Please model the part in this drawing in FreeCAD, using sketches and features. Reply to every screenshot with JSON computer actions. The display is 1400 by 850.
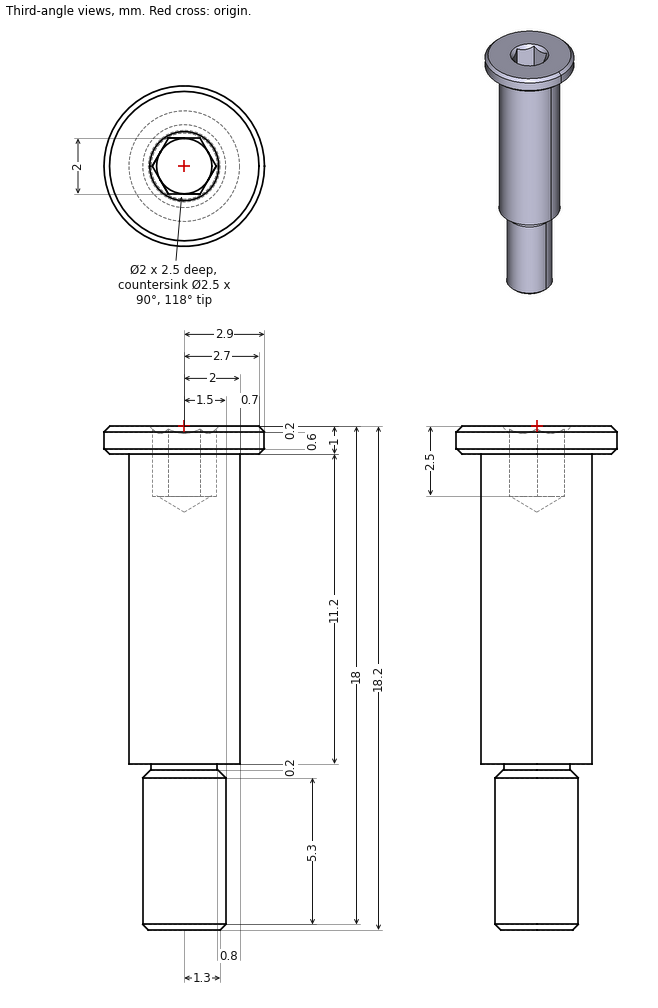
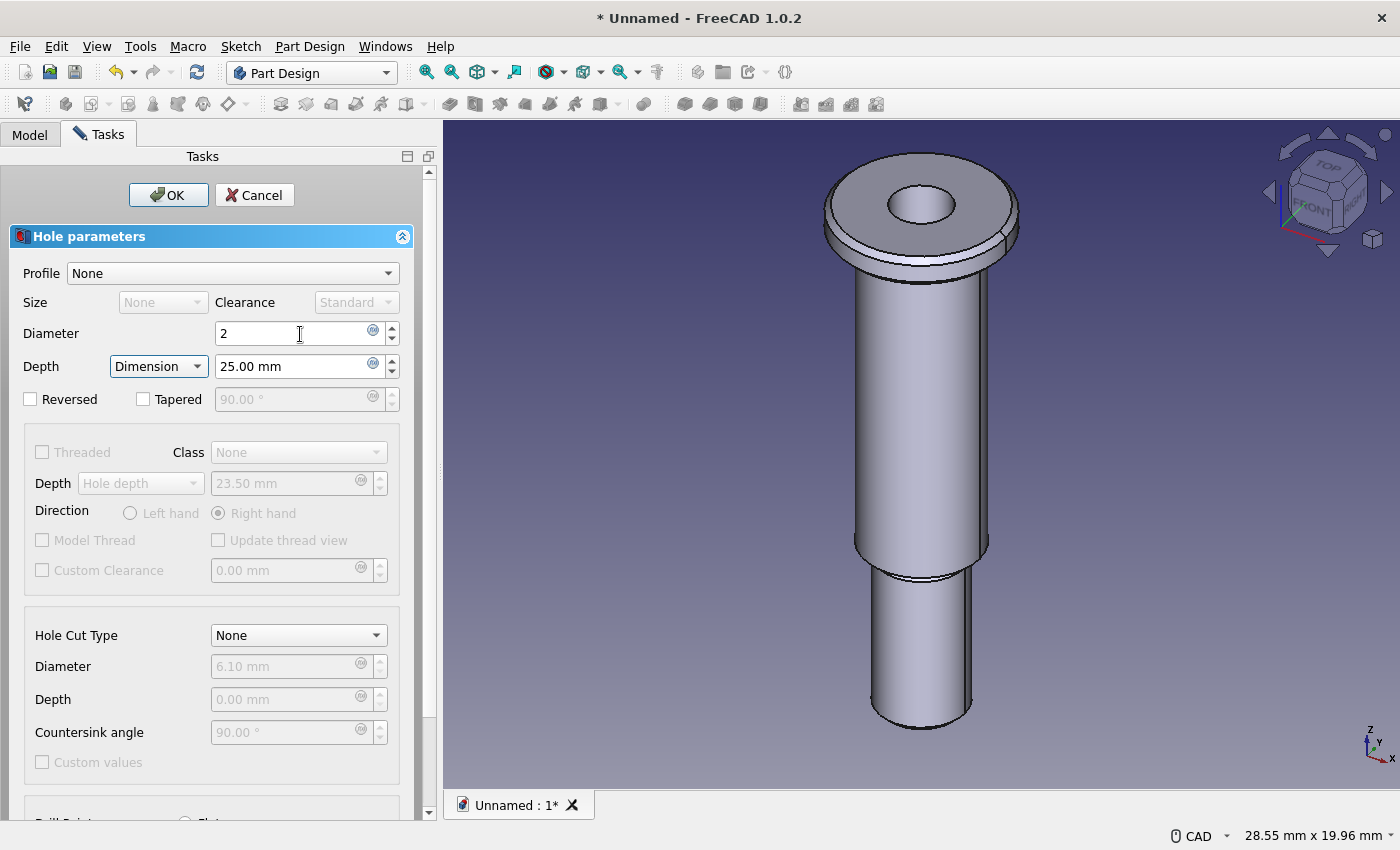
{"action": "triple_click", "coordinate": [300, 366]}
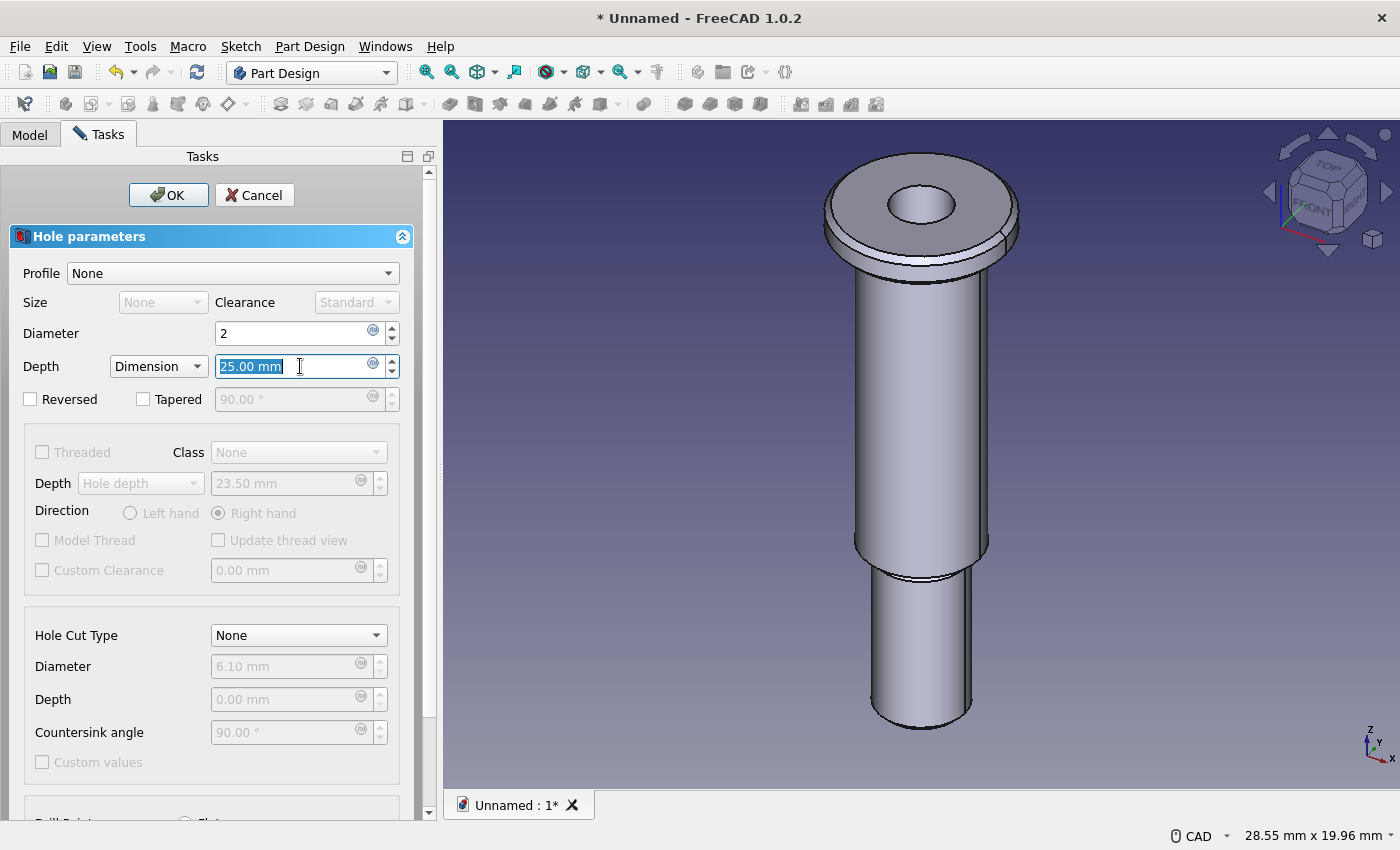
{"action": "type", "text": "2.5"}
{"action": "key", "text": "Tab"}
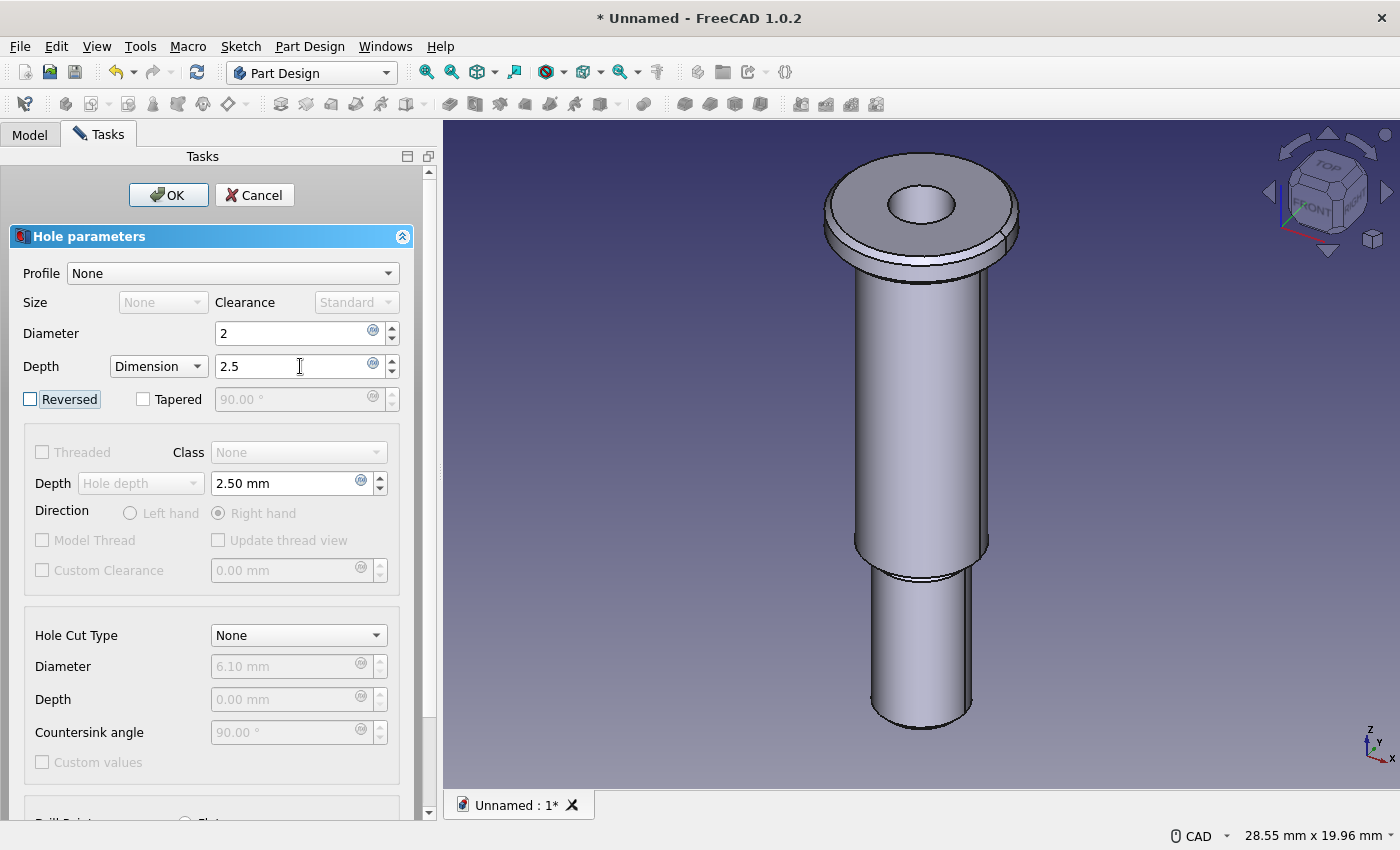
{"action": "left_click", "coordinate": [300, 636]}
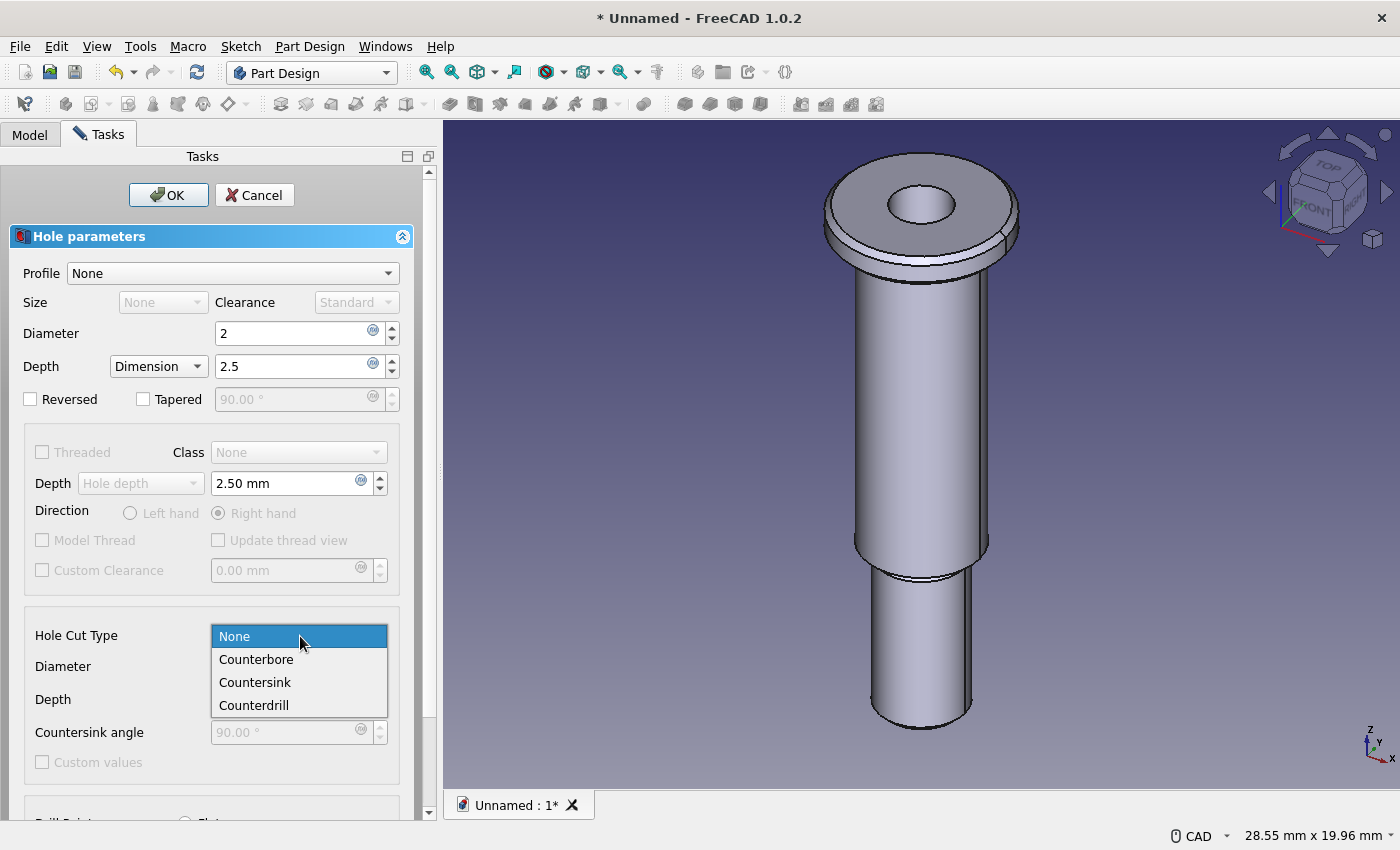
{"action": "left_click", "coordinate": [298, 682]}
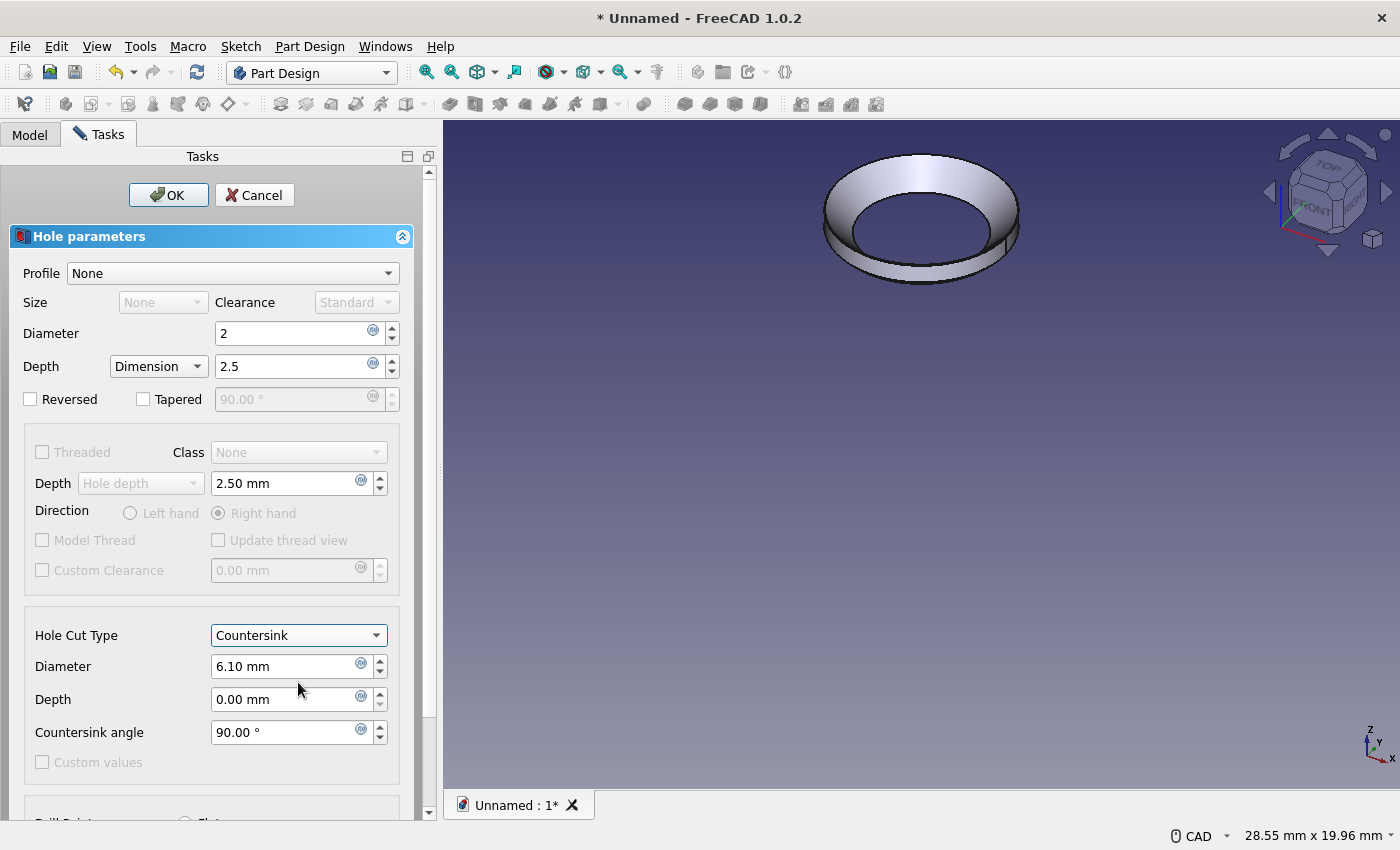
{"action": "triple_click", "coordinate": [292, 666]}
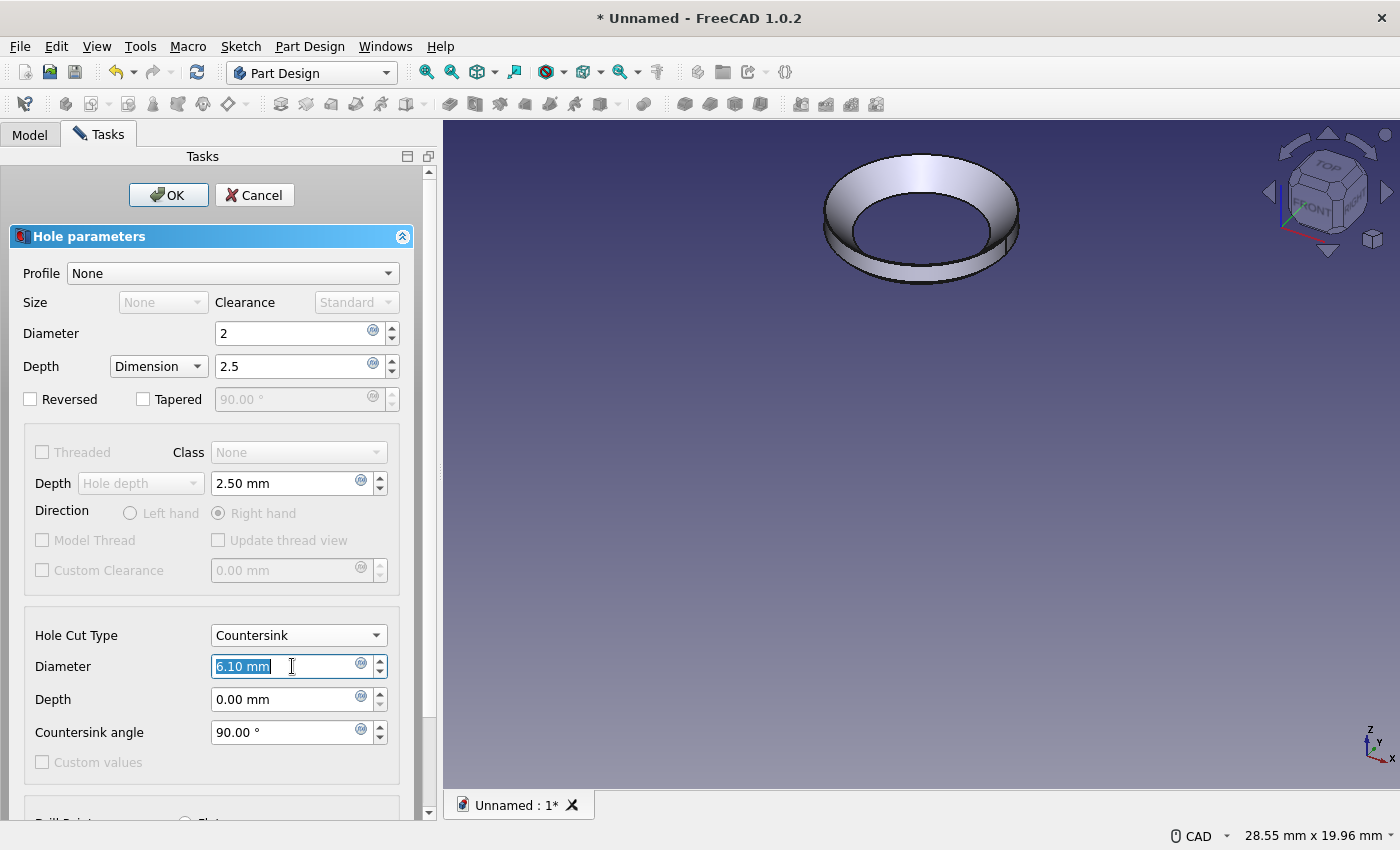
{"action": "type", "text": "2.5"}
{"action": "key", "text": "Tab"}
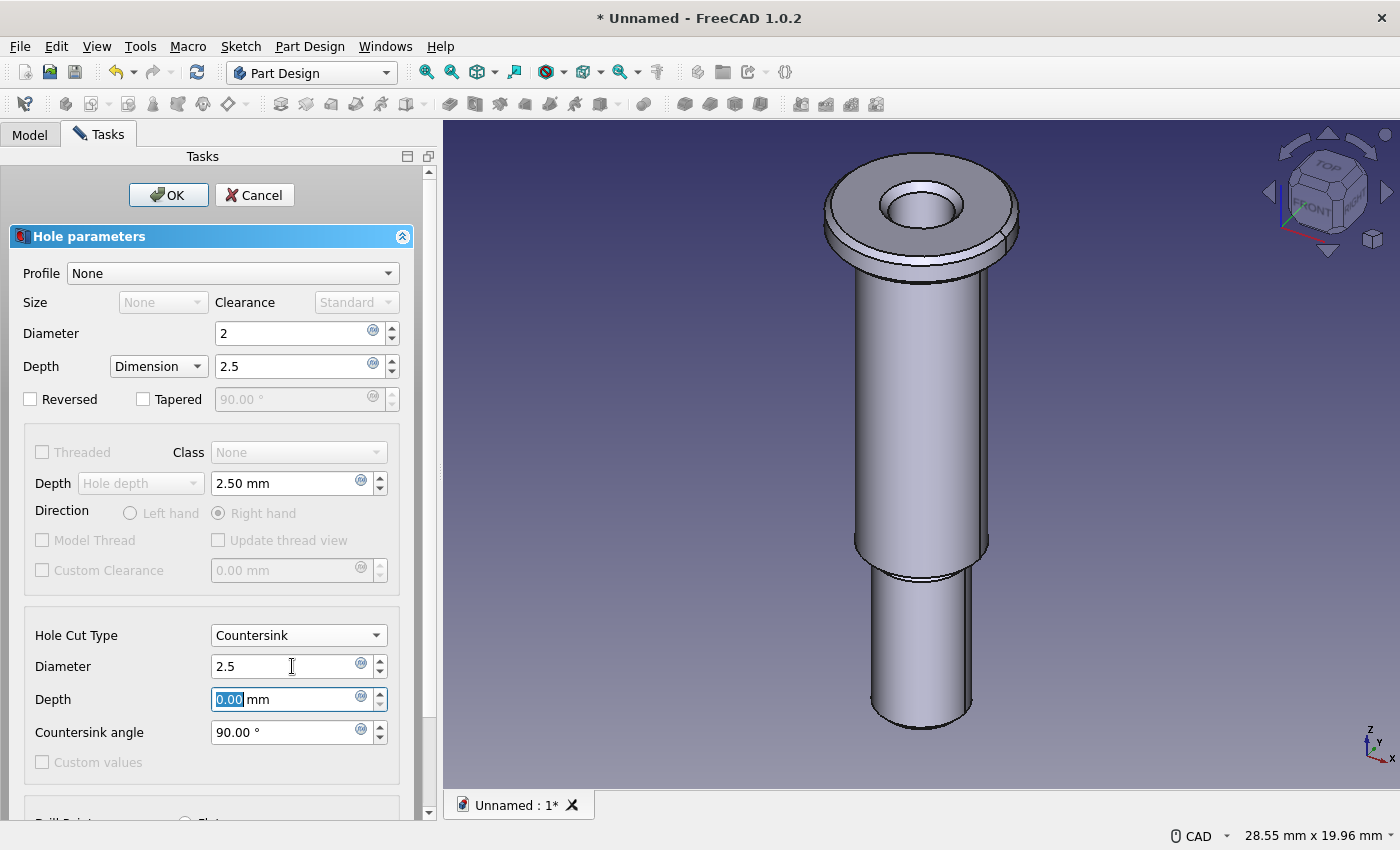
{"action": "left_click", "coordinate": [169, 195]}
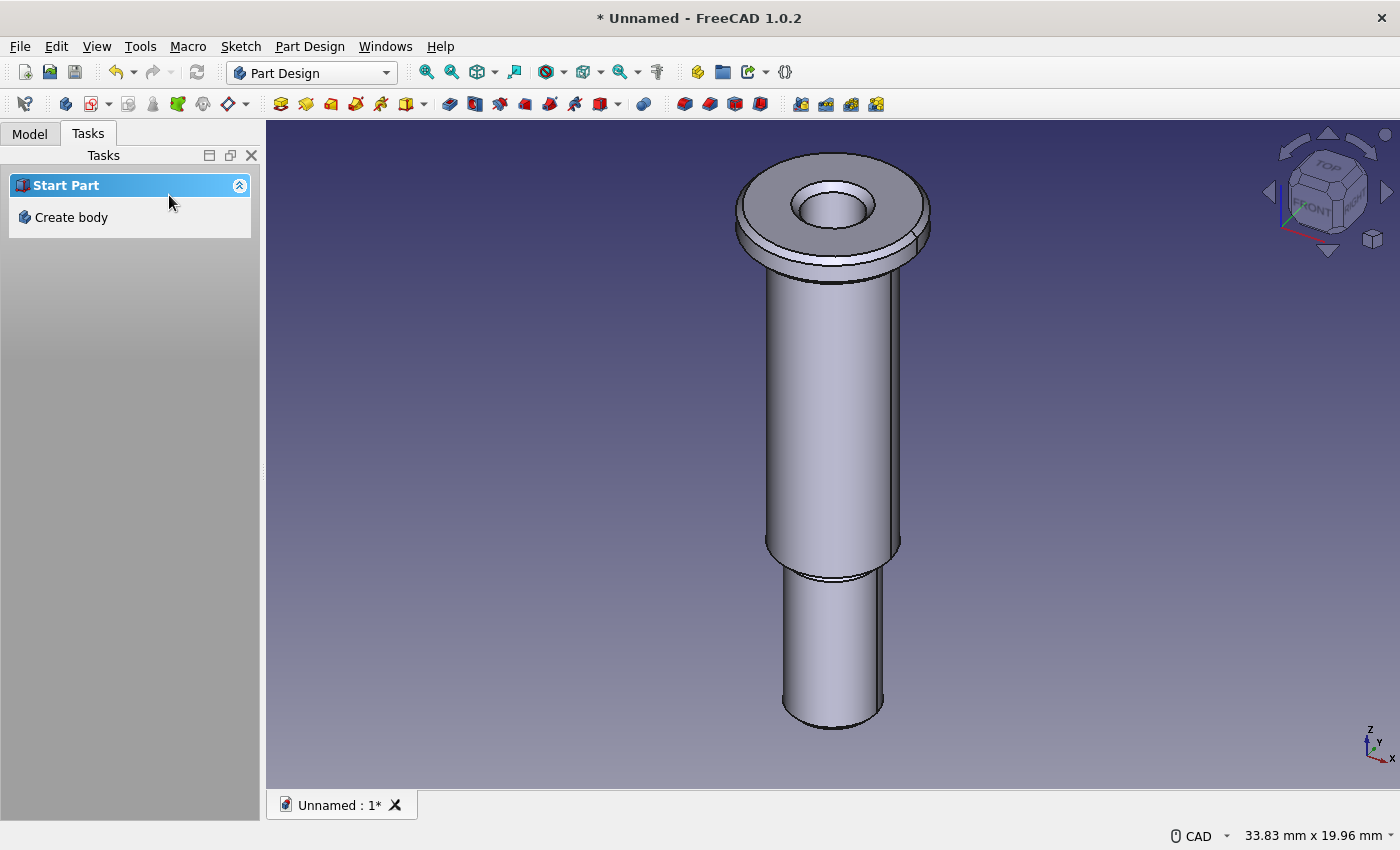
{"action": "left_click", "coordinate": [90, 104]}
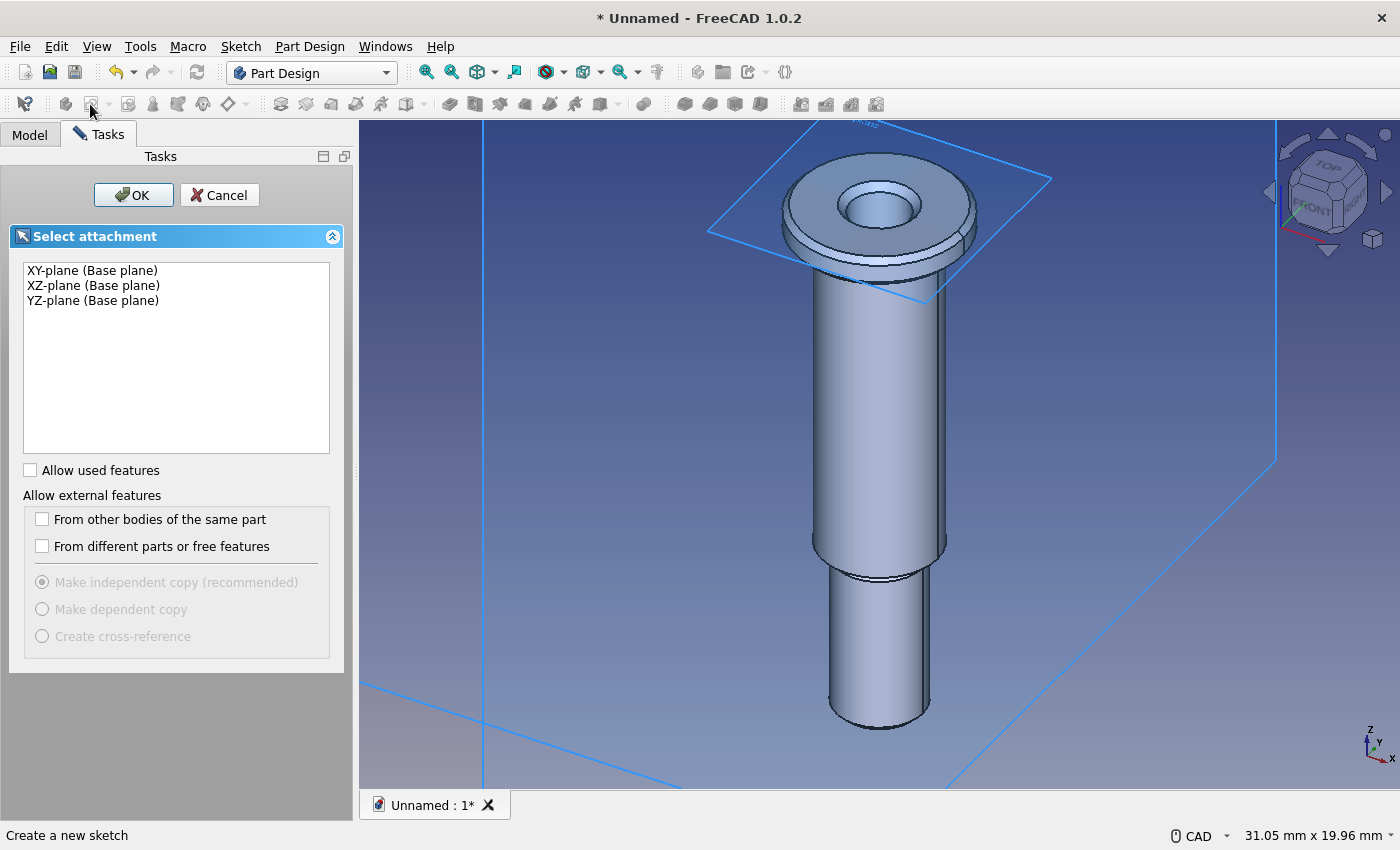
{"action": "left_click", "coordinate": [84, 270]}